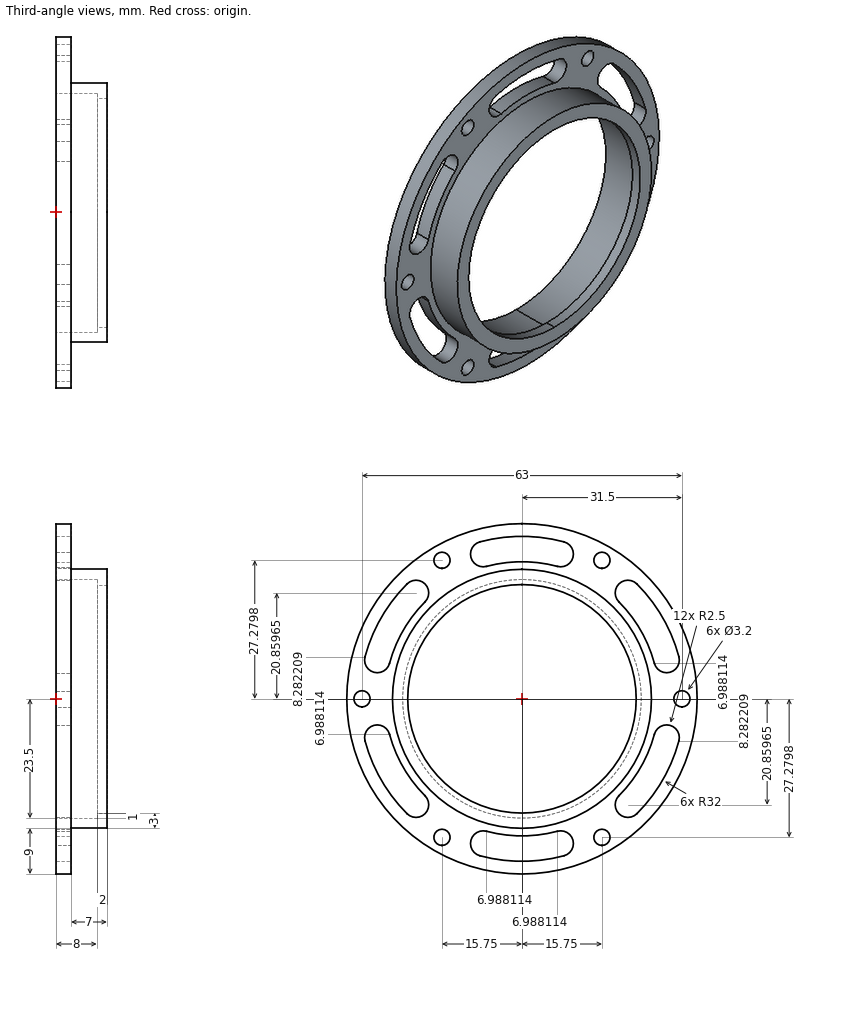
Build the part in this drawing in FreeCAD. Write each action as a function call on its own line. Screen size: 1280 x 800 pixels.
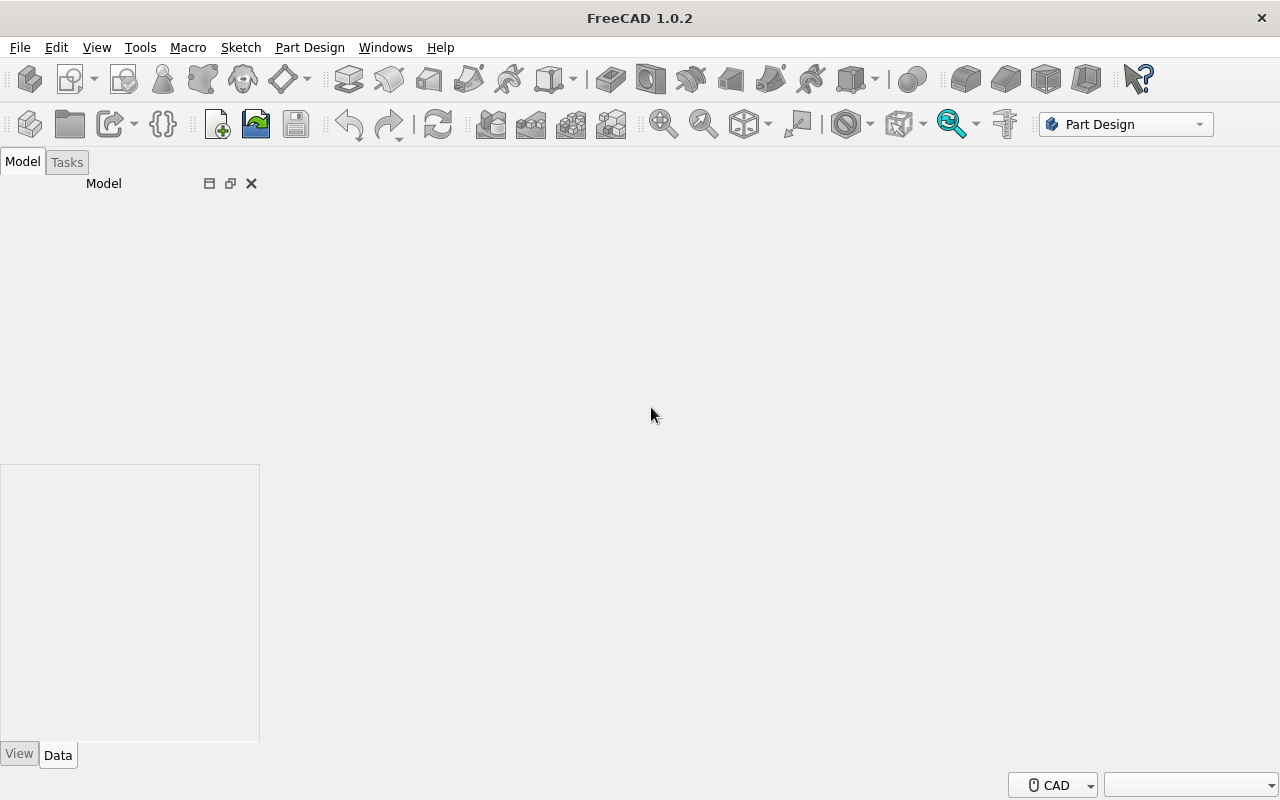
key(ctrl+n)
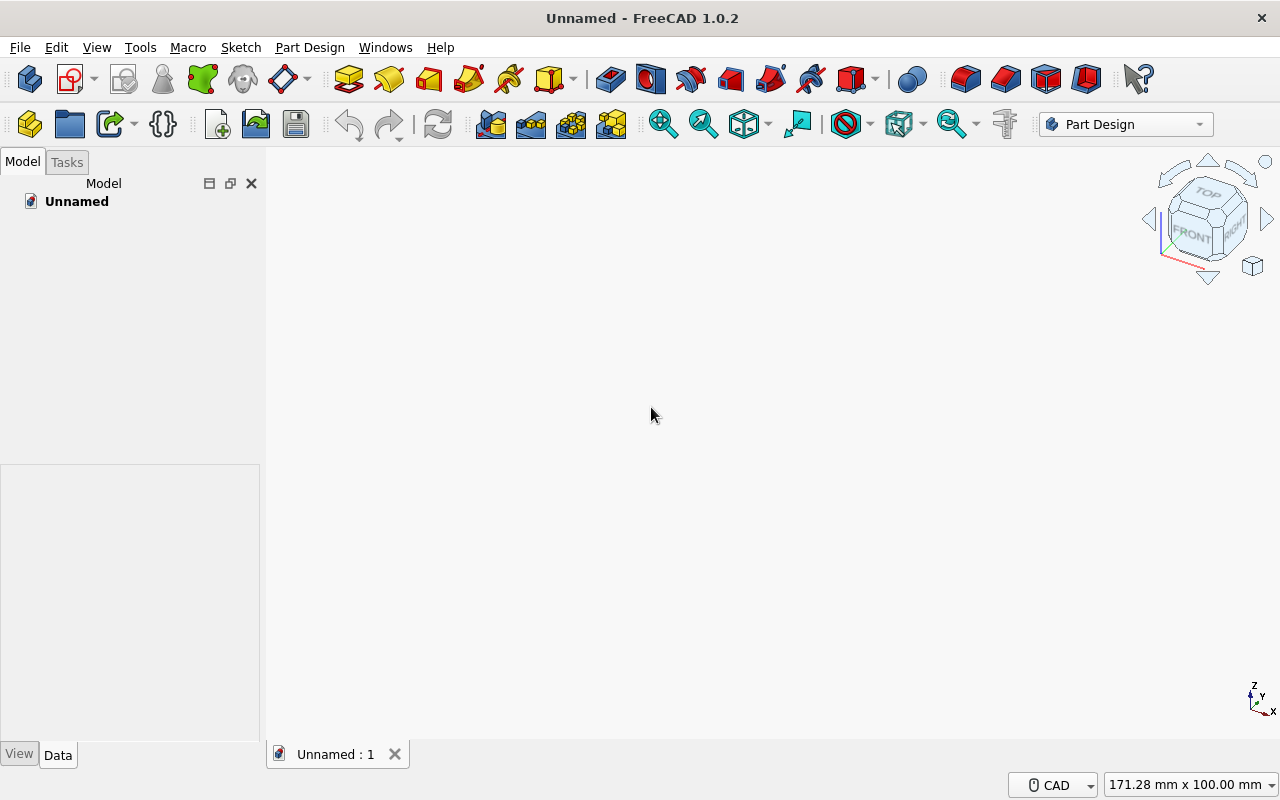
click(70, 80)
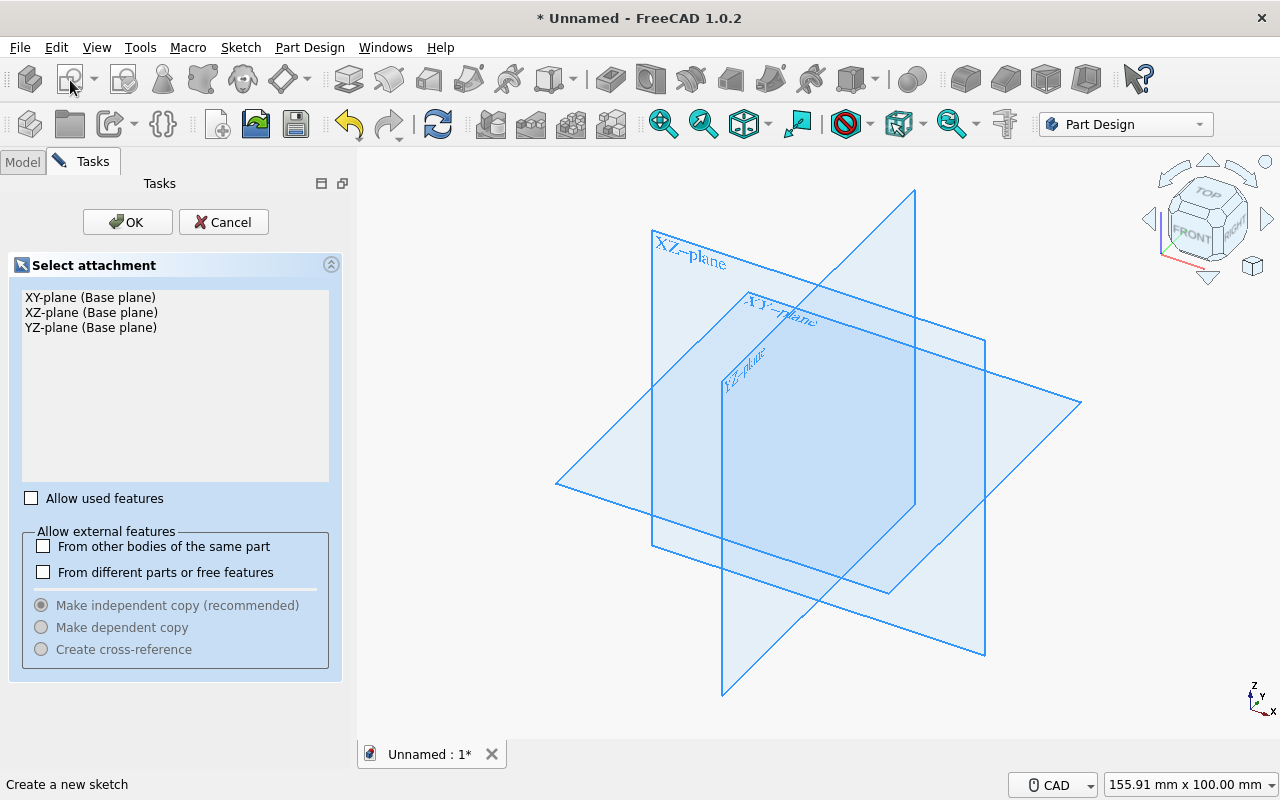
click(82, 312)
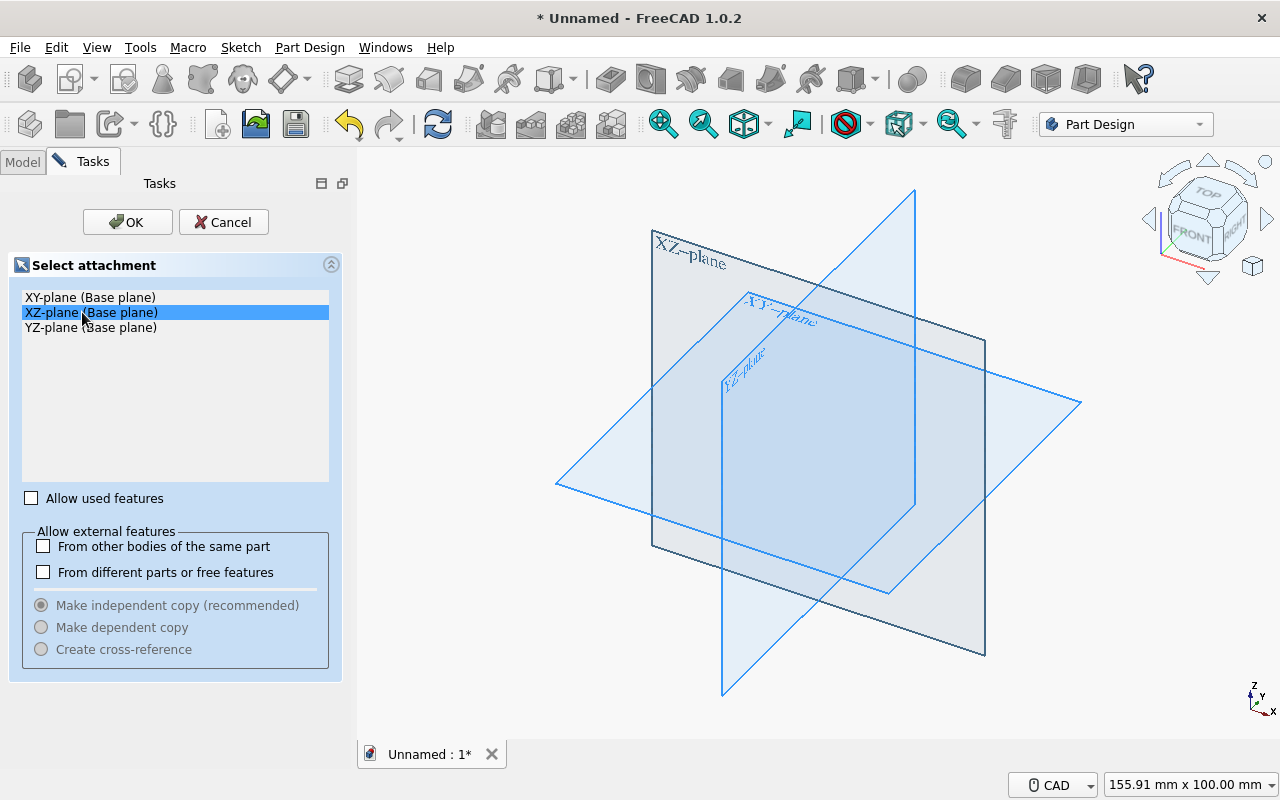
click(128, 222)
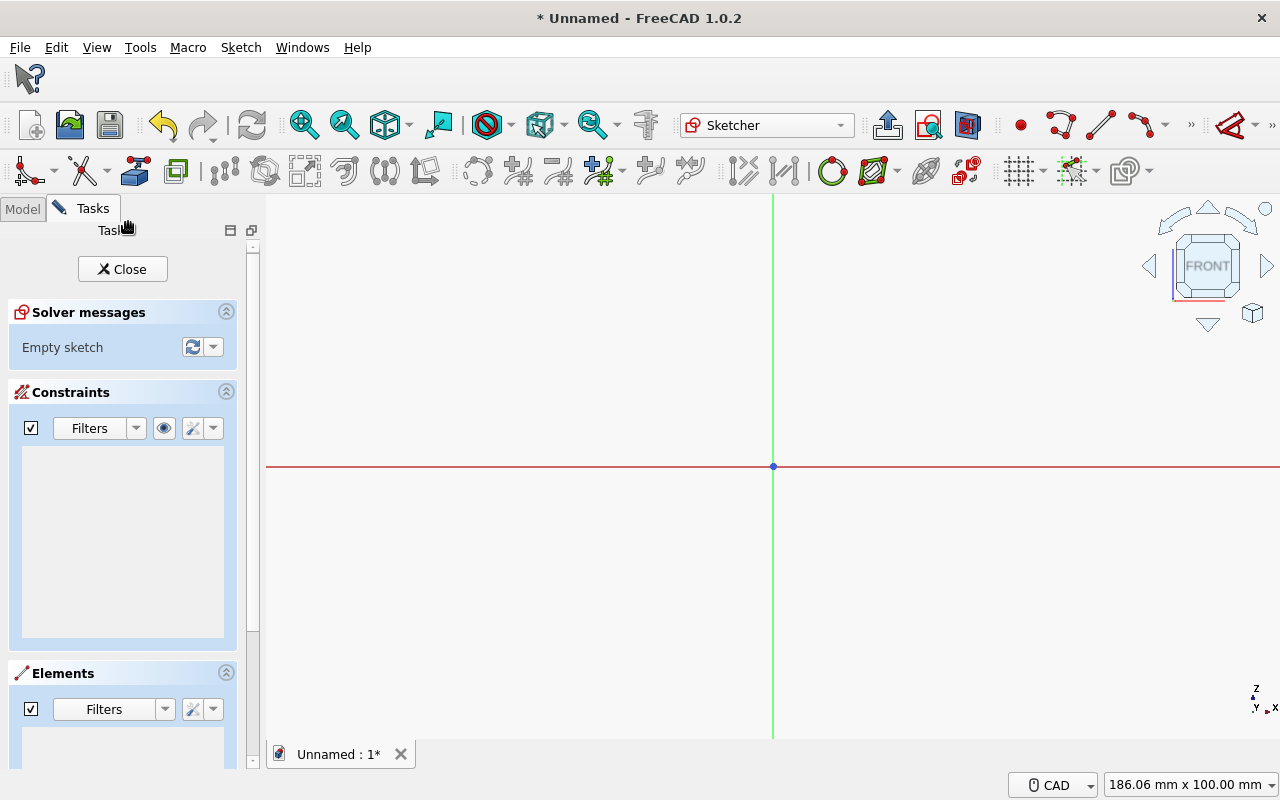
scroll(824, 661, up, 8)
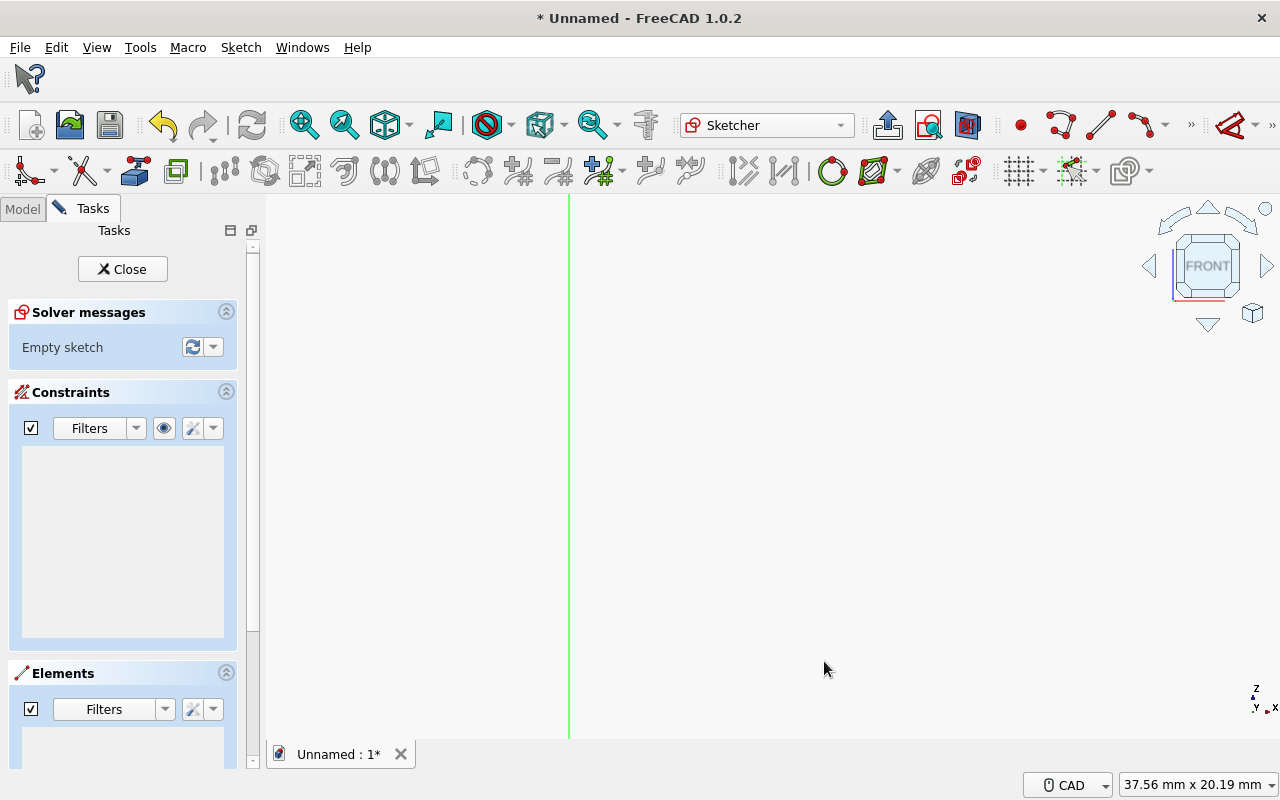
click(1062, 126)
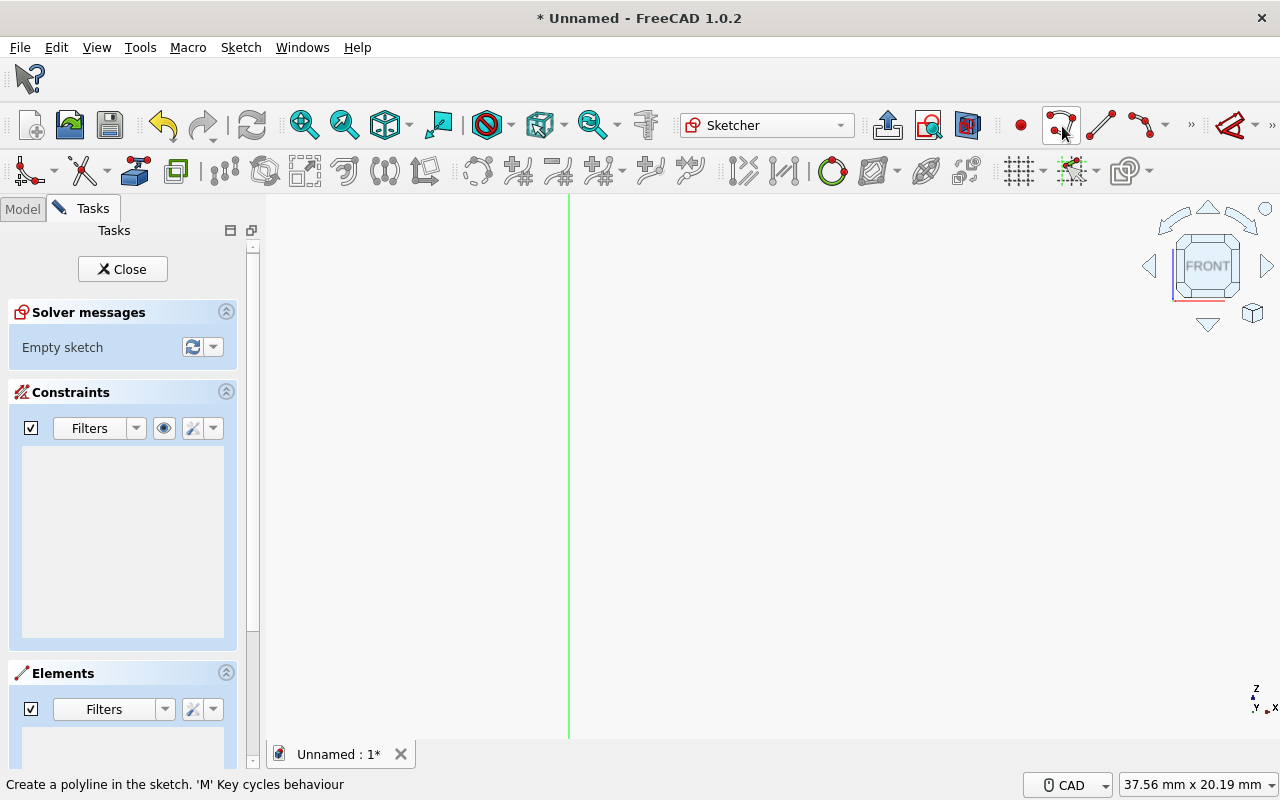
click(569, 329)
click(785, 329)
click(785, 302)
click(839, 302)
click(839, 383)
click(650, 383)
click(650, 626)
click(578, 626)
click(569, 330)
key(Escape)
key(Escape)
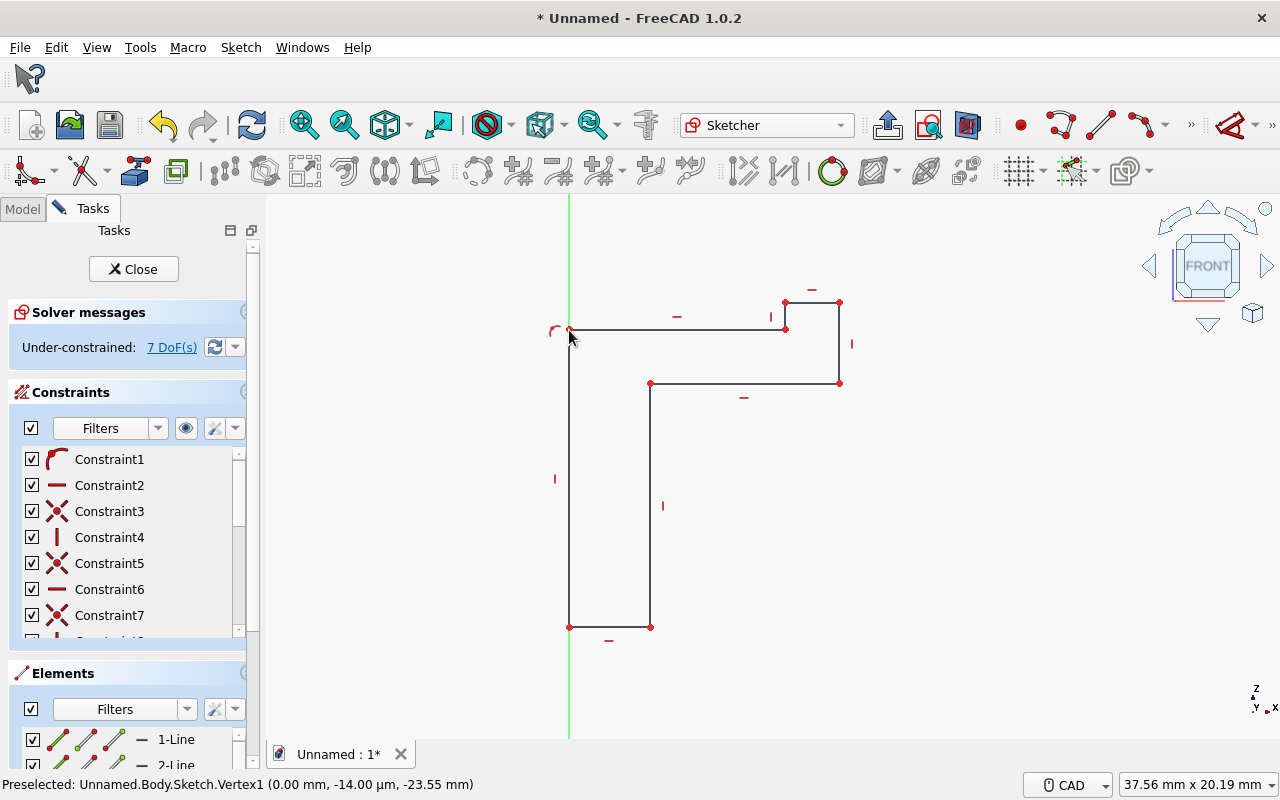
key(d)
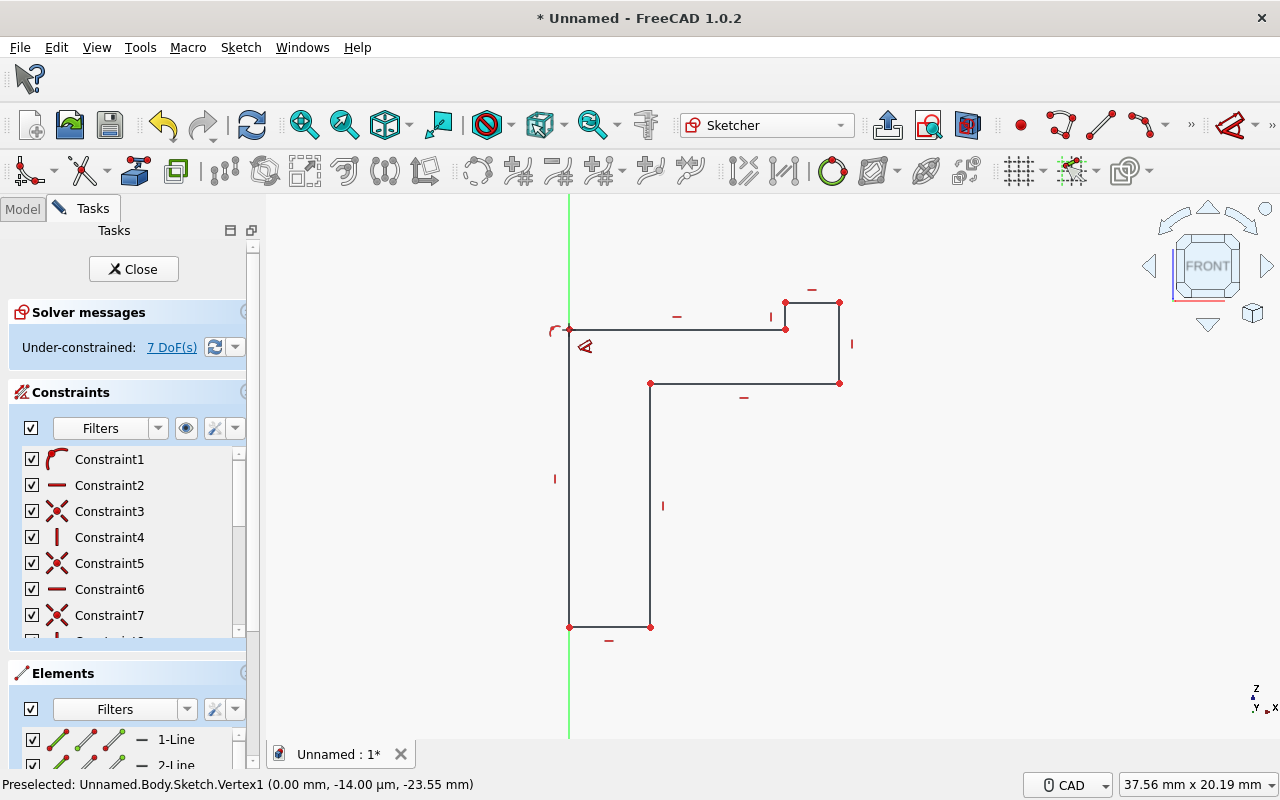
click(634, 330)
click(677, 296)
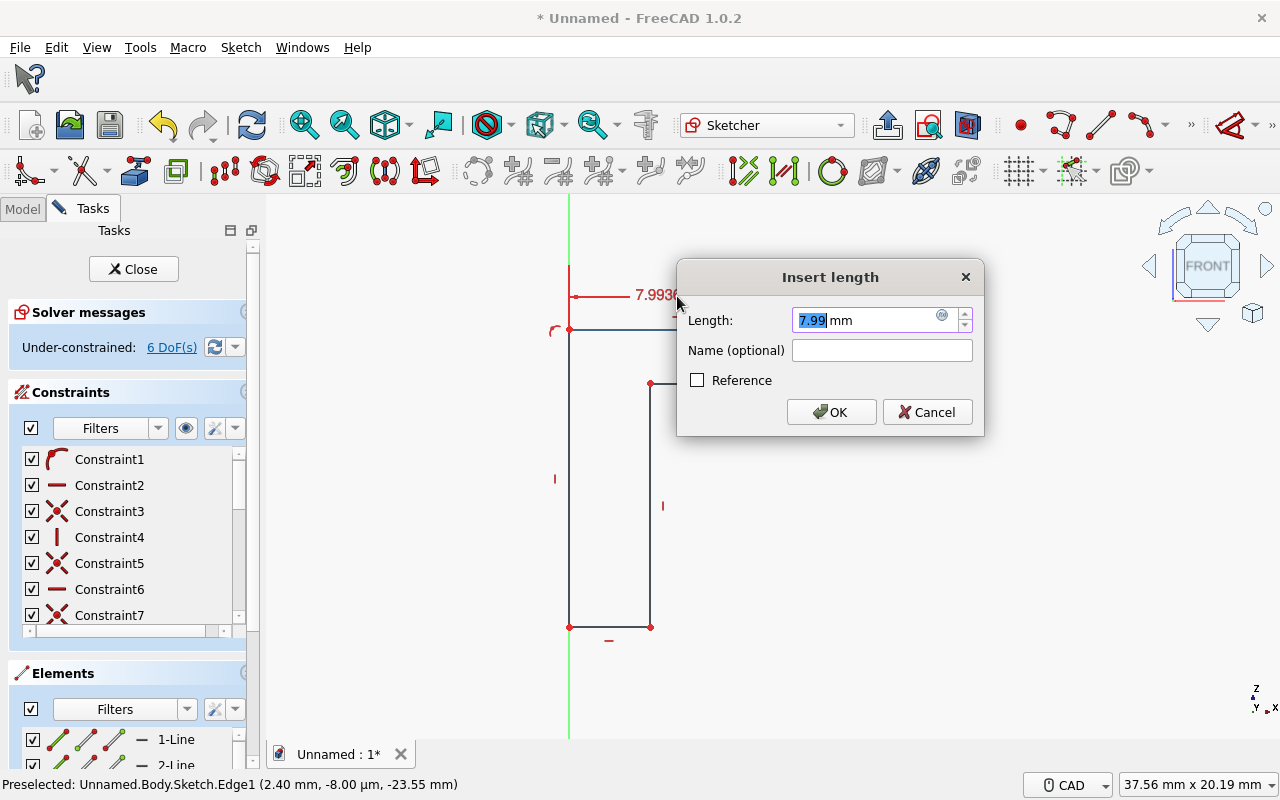
text(8)
key(Return)